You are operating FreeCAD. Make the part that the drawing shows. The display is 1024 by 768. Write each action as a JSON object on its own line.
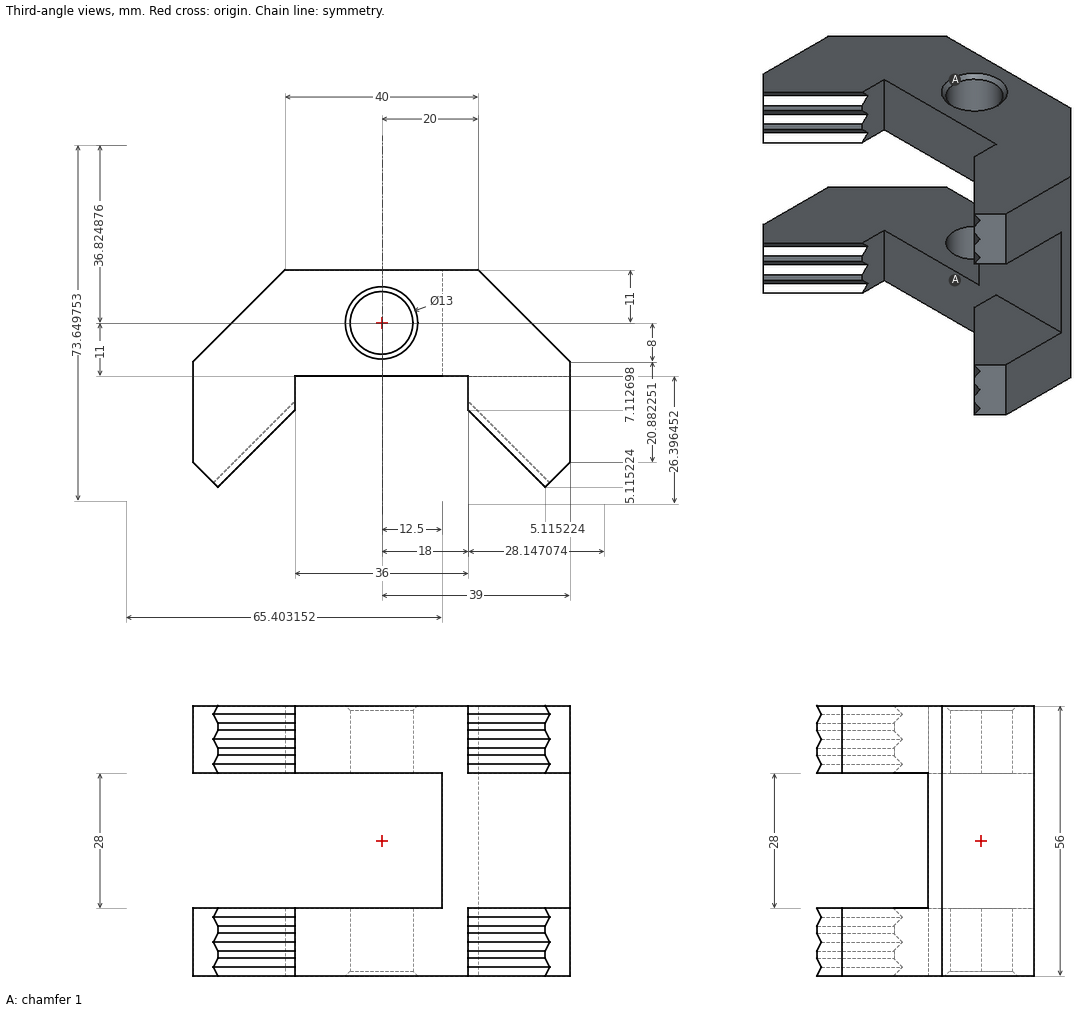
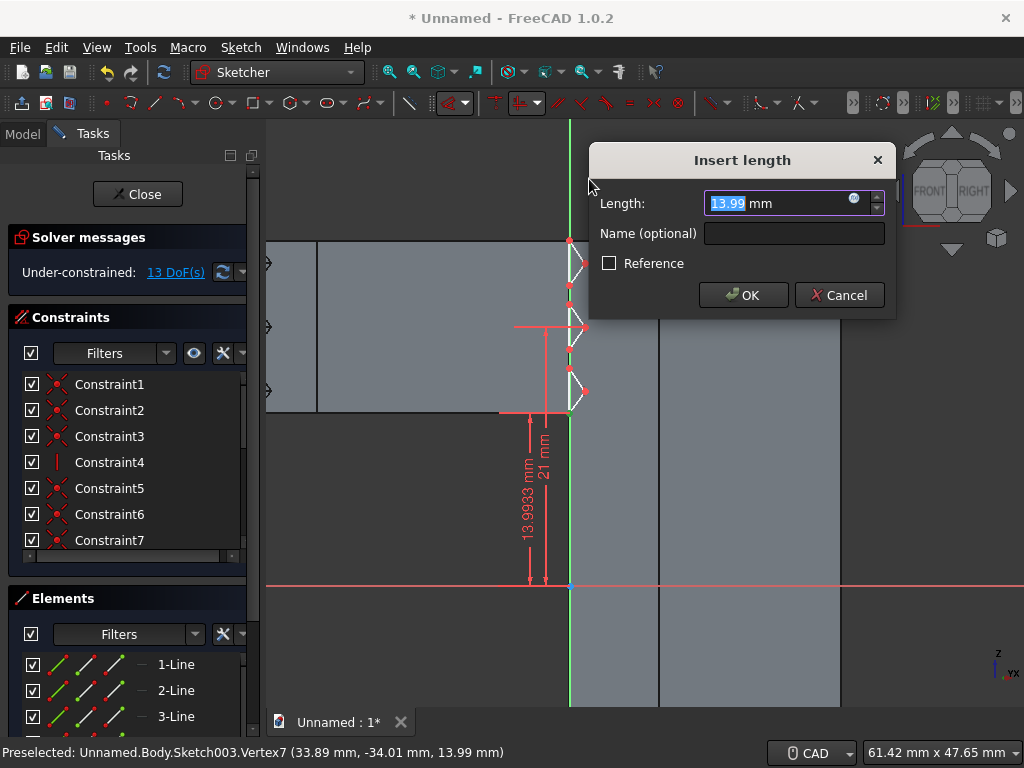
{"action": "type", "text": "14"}
{"action": "key", "text": "Return"}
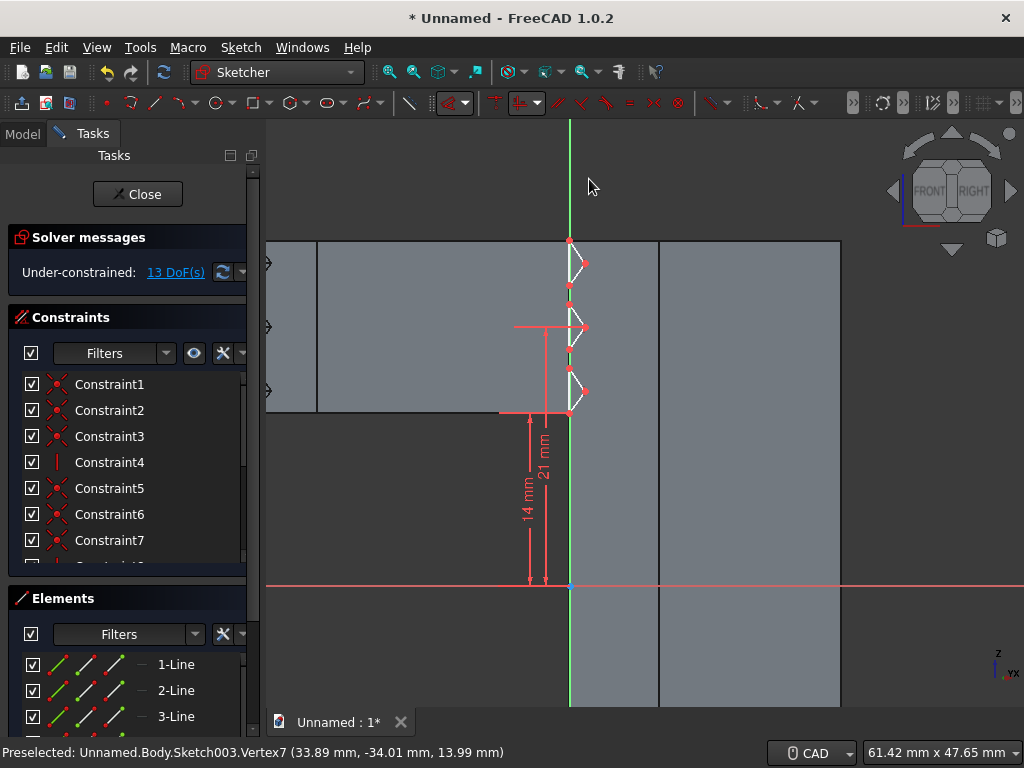
{"action": "left_click", "coordinate": [569, 241]}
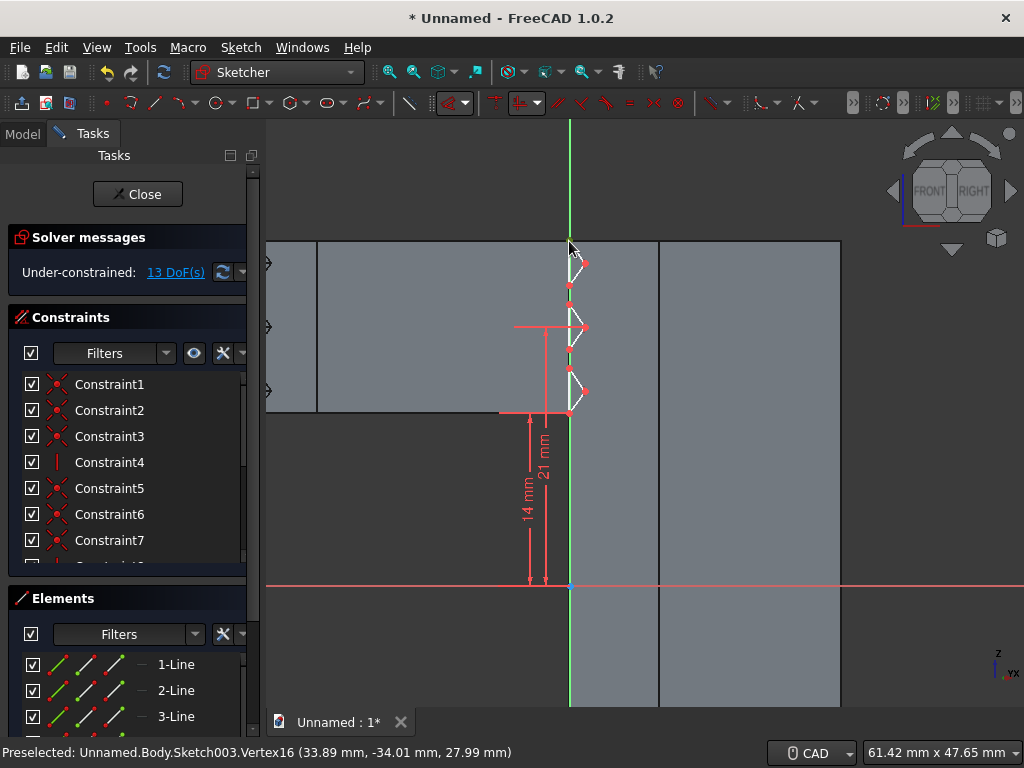
{"action": "left_click", "coordinate": [468, 104]}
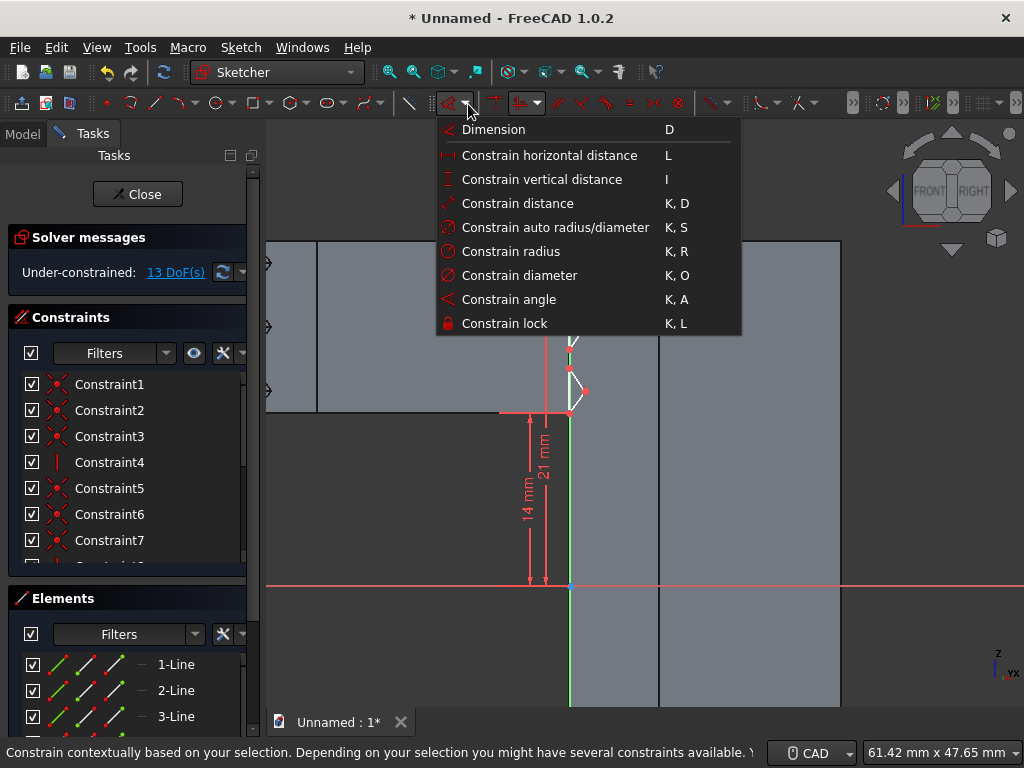
{"action": "left_click", "coordinate": [589, 179]}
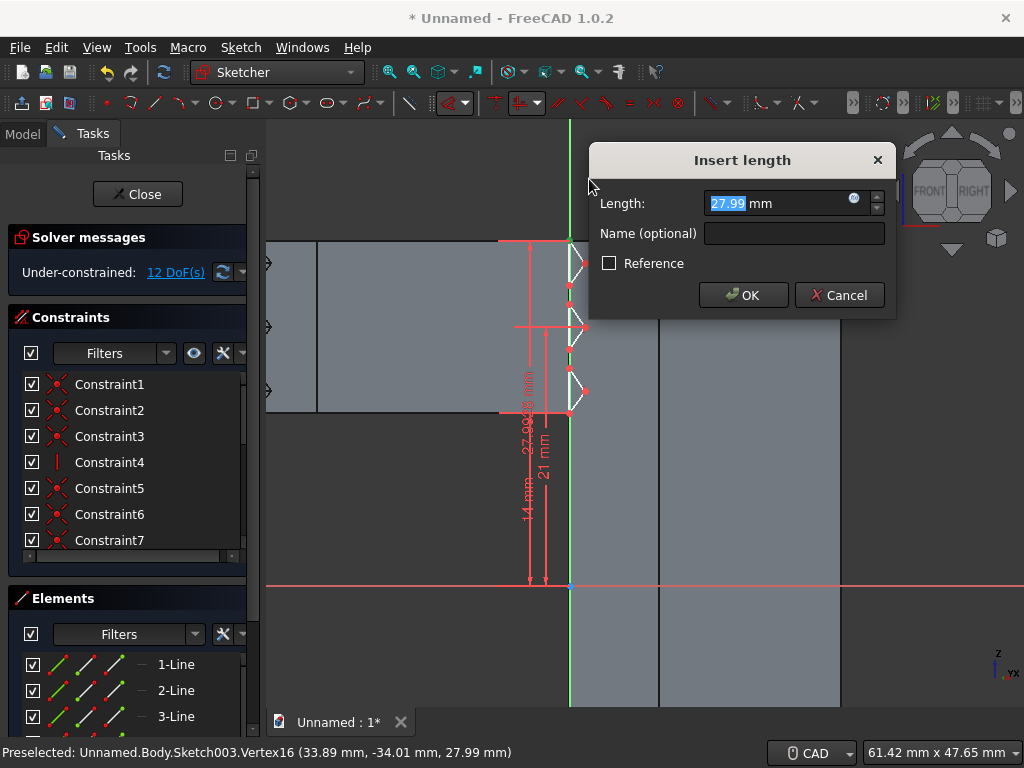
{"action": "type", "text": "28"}
{"action": "key", "text": "Return"}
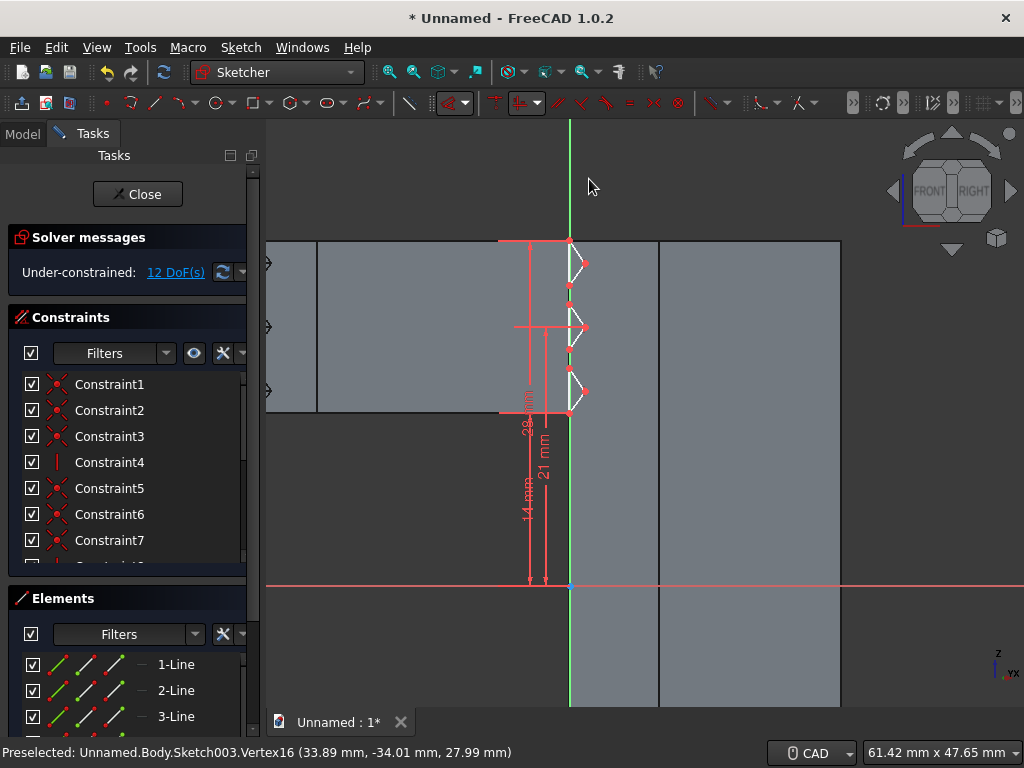
{"action": "scroll", "coordinate": [569, 323], "scroll_direction": "up", "scroll_amount": 2}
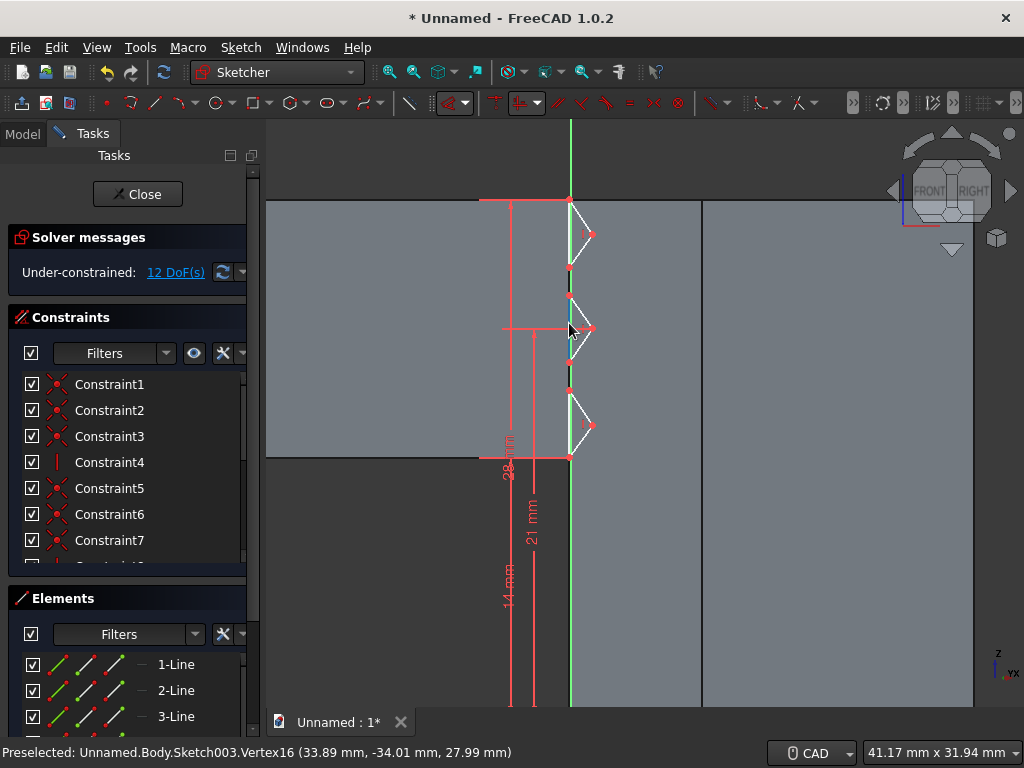
{"action": "left_click", "coordinate": [569, 322]}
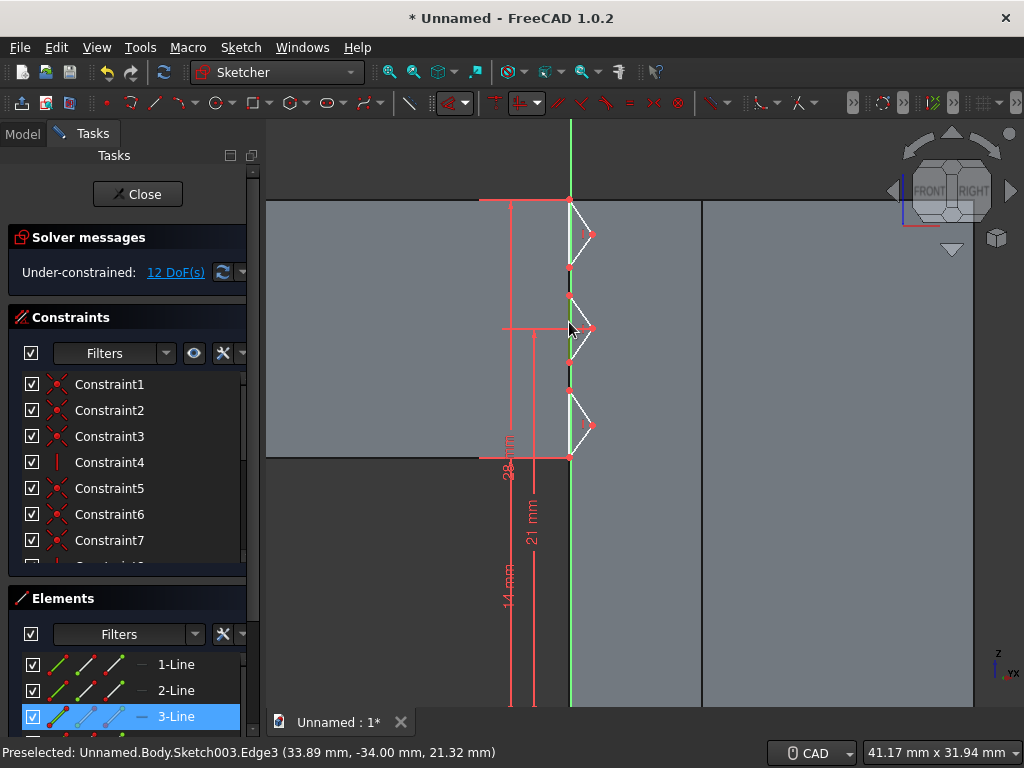
{"action": "left_click", "coordinate": [468, 104]}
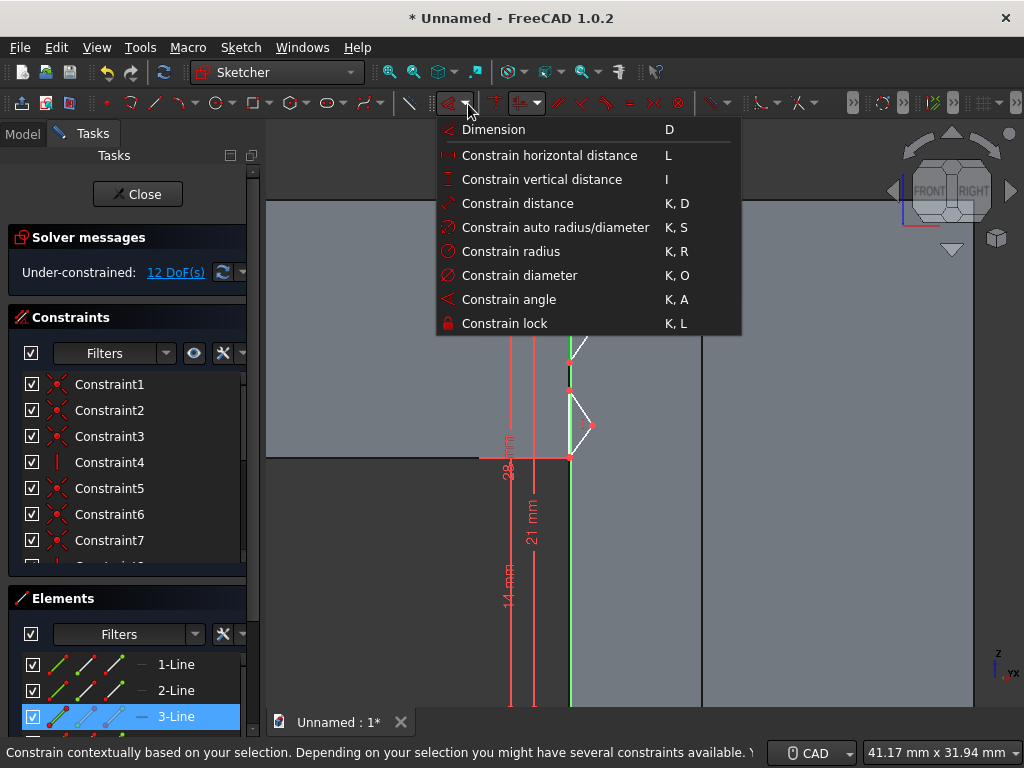
{"action": "left_click", "coordinate": [589, 179]}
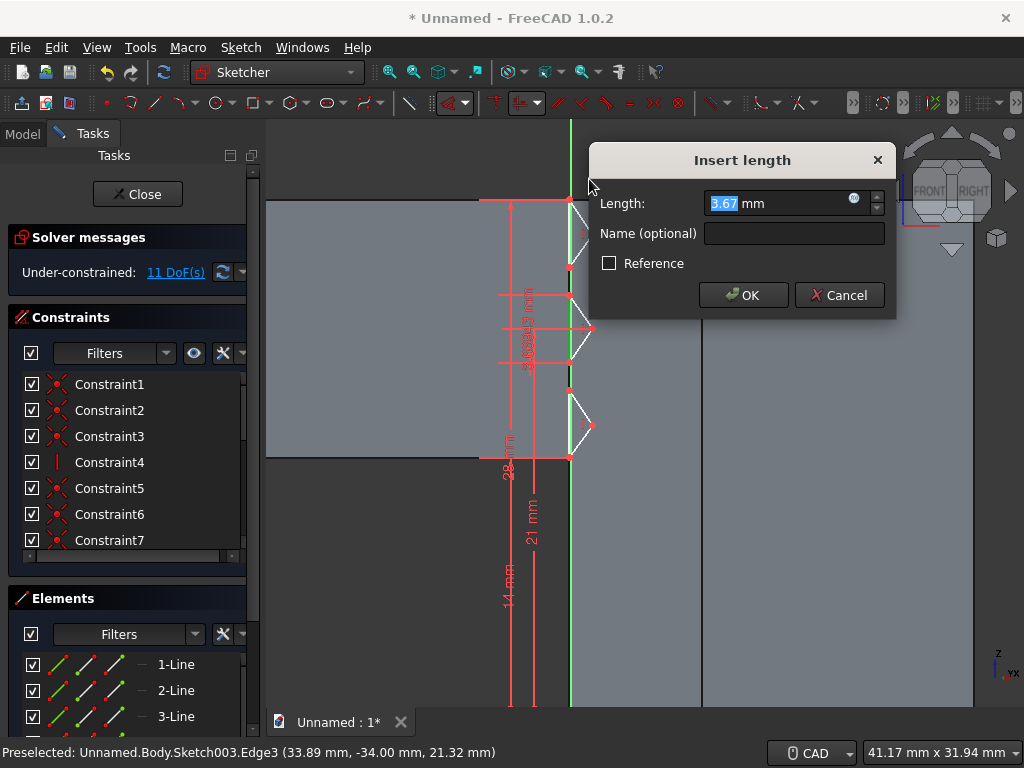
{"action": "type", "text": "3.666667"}
{"action": "key", "text": "Return"}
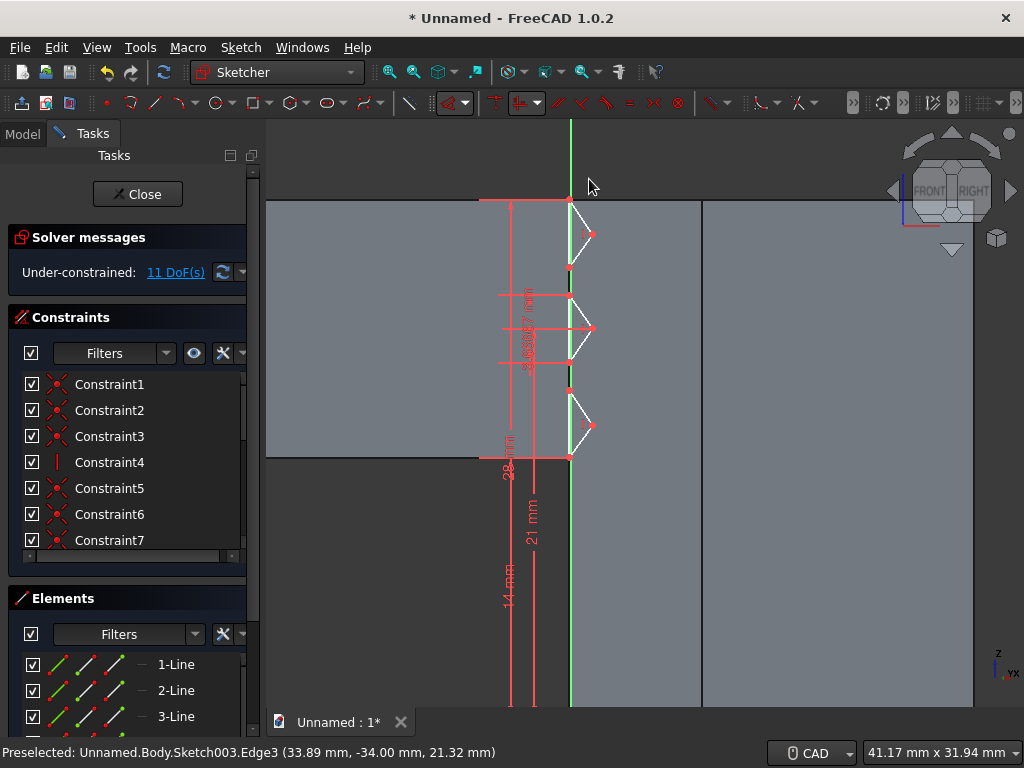
{"action": "scroll", "coordinate": [569, 410], "scroll_direction": "up", "scroll_amount": 2}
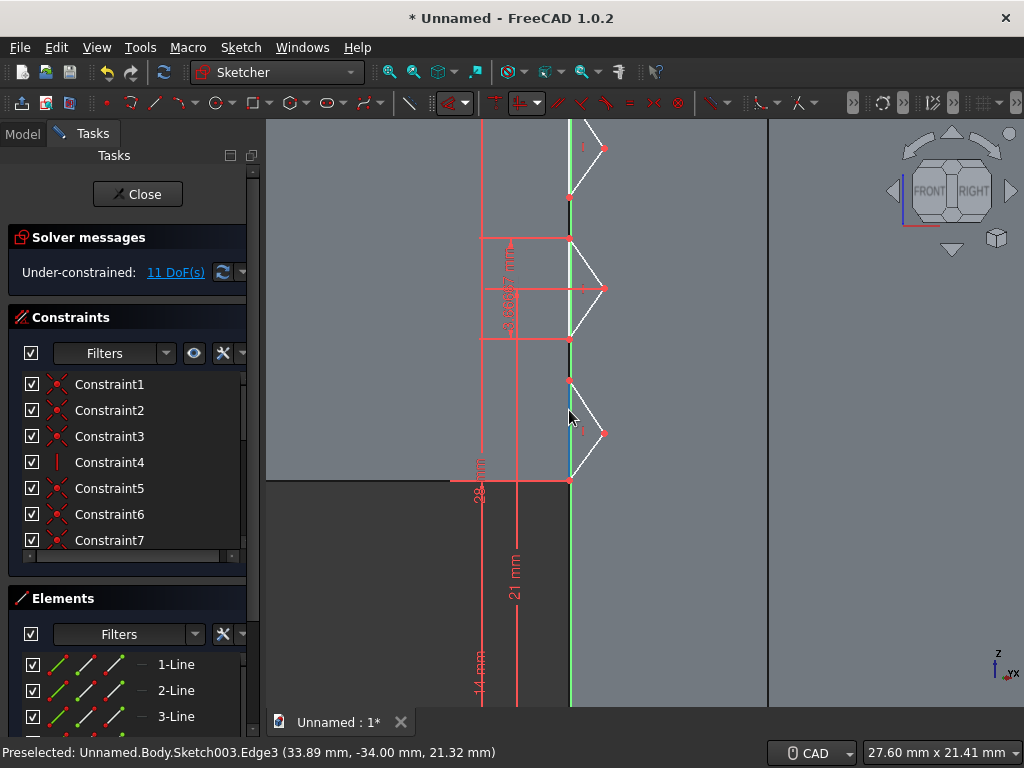
{"action": "left_click", "coordinate": [569, 411]}